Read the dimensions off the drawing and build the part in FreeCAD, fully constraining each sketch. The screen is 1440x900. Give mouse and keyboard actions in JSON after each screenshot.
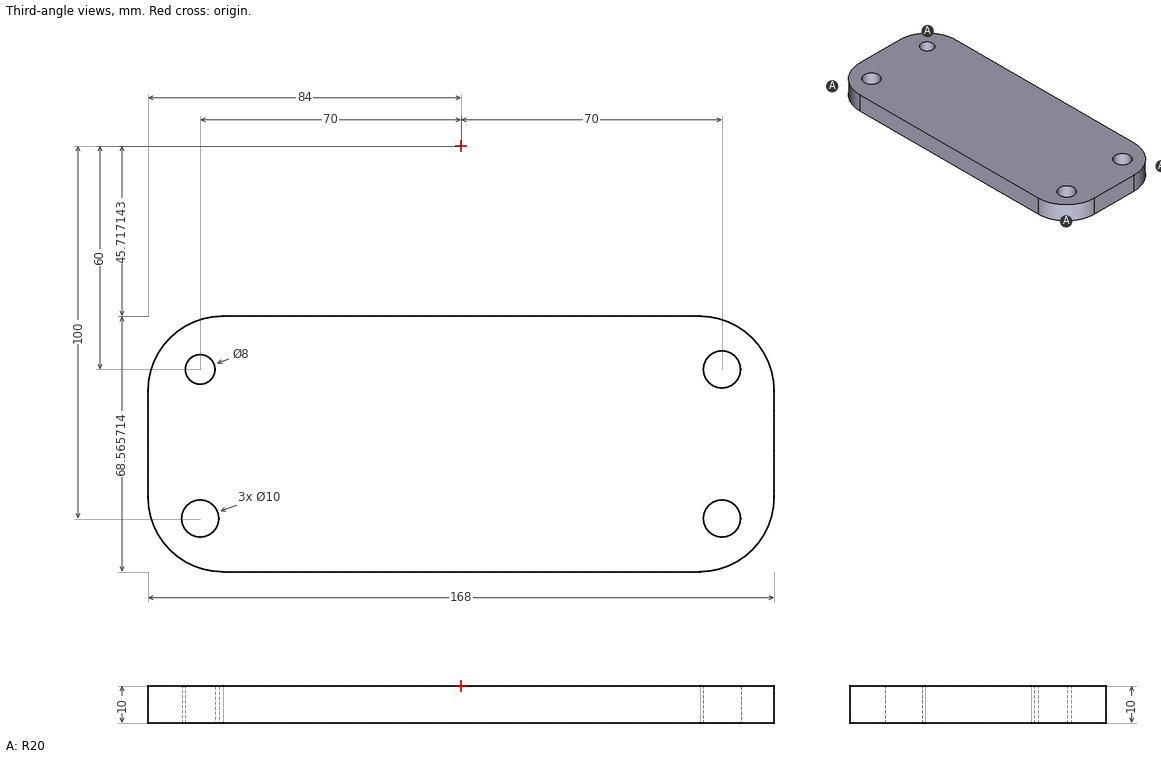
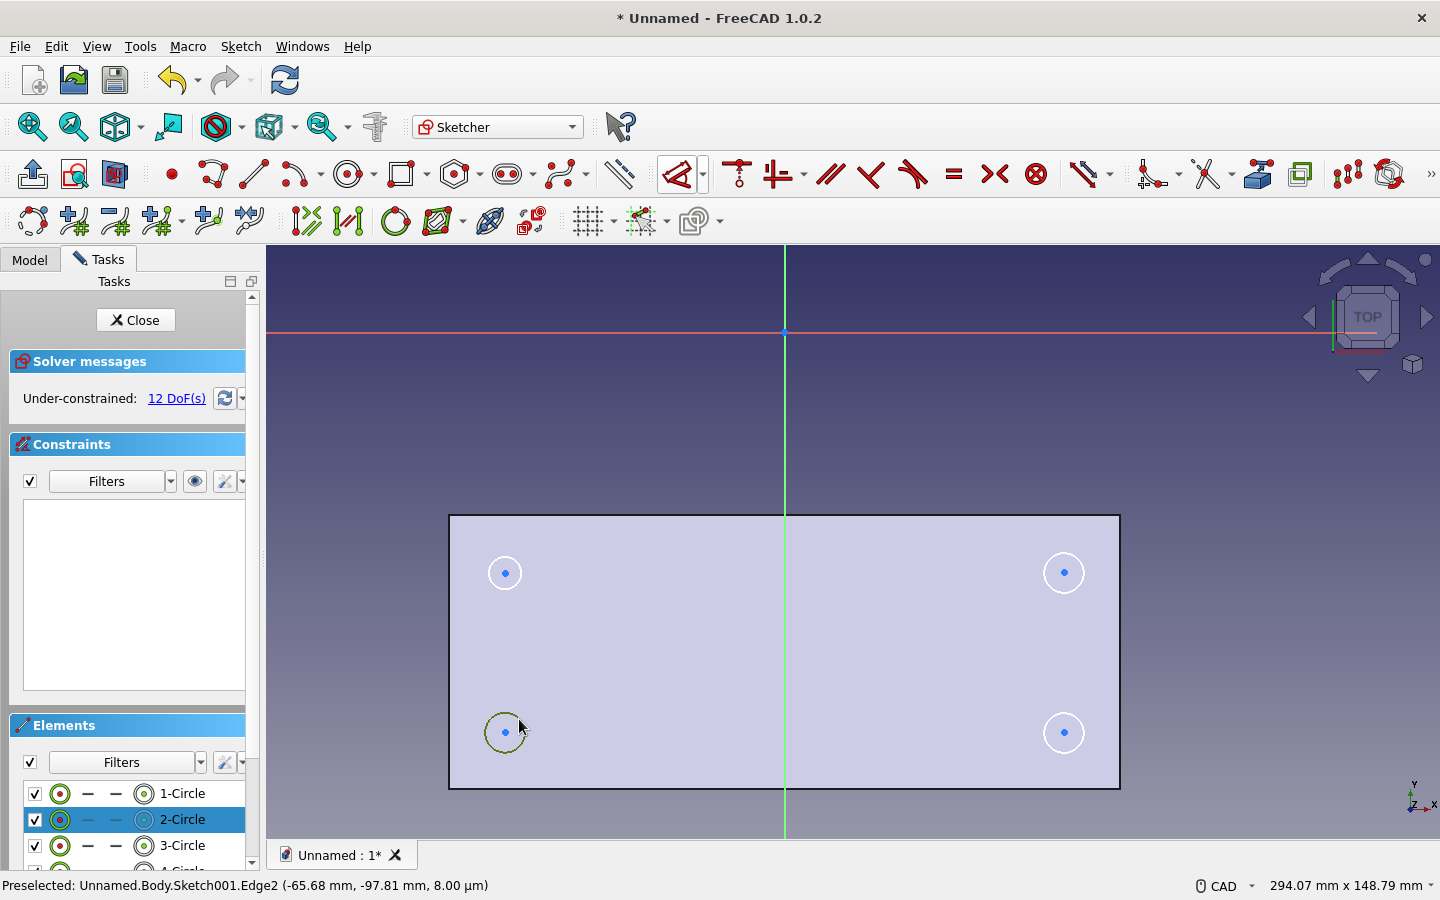
{"action": "left_click", "coordinate": [1078, 559]}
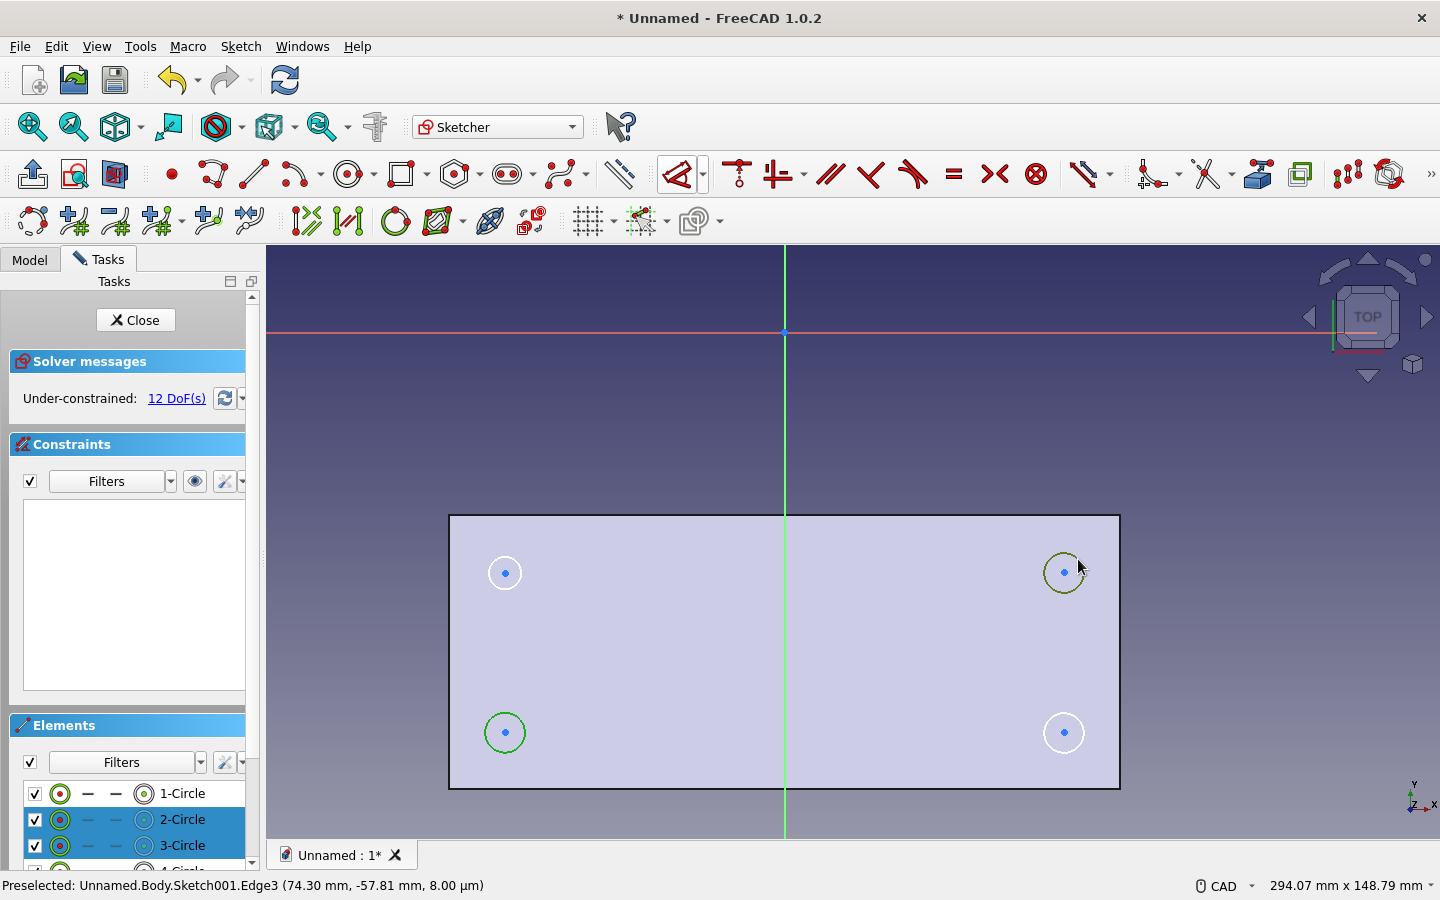
{"action": "left_click", "coordinate": [1078, 719]}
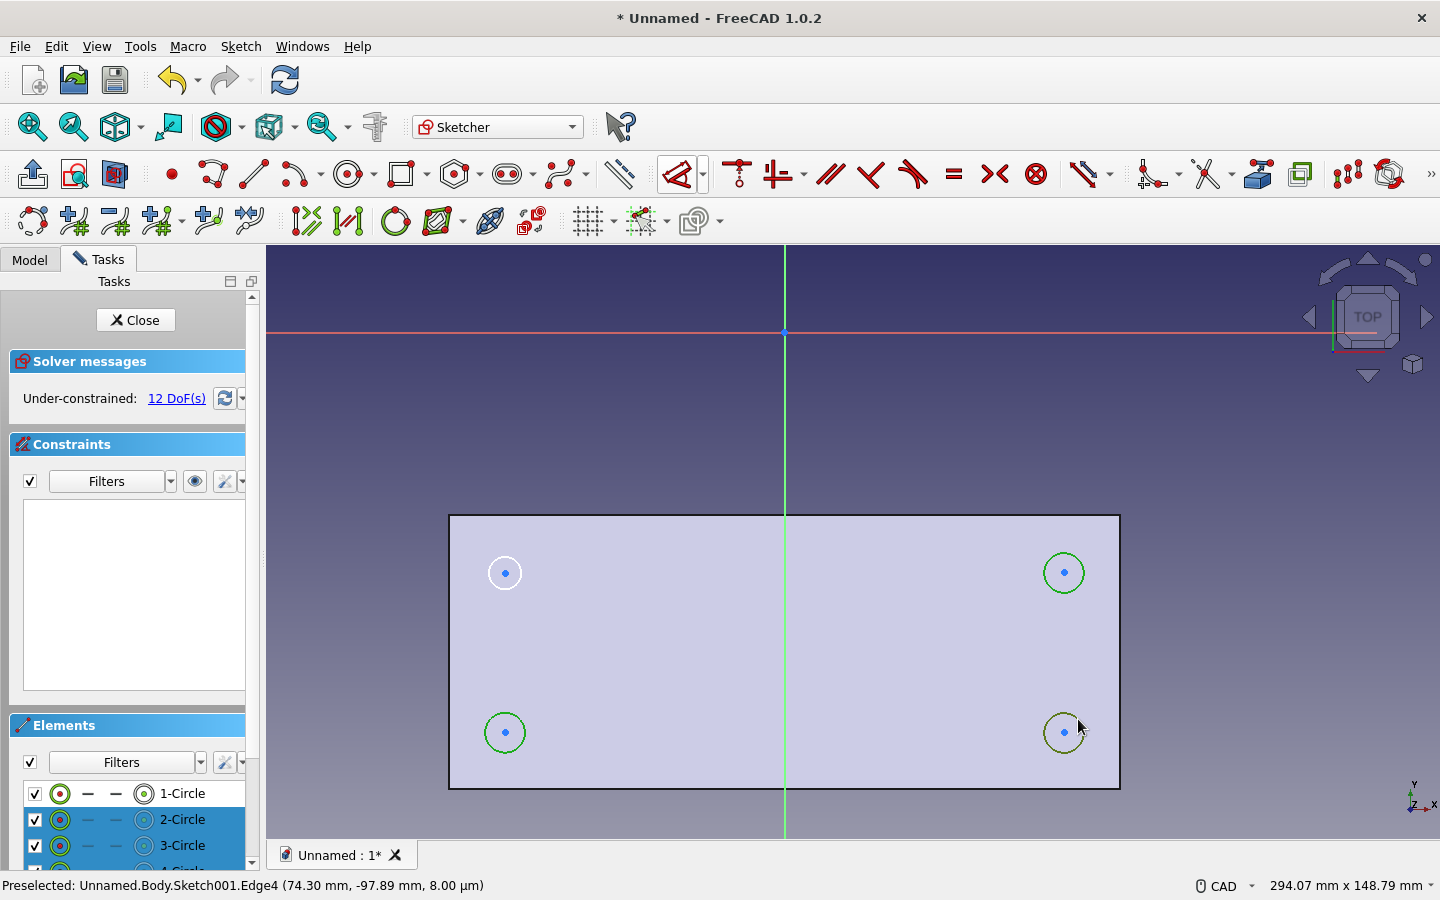
{"action": "left_click", "coordinate": [954, 174]}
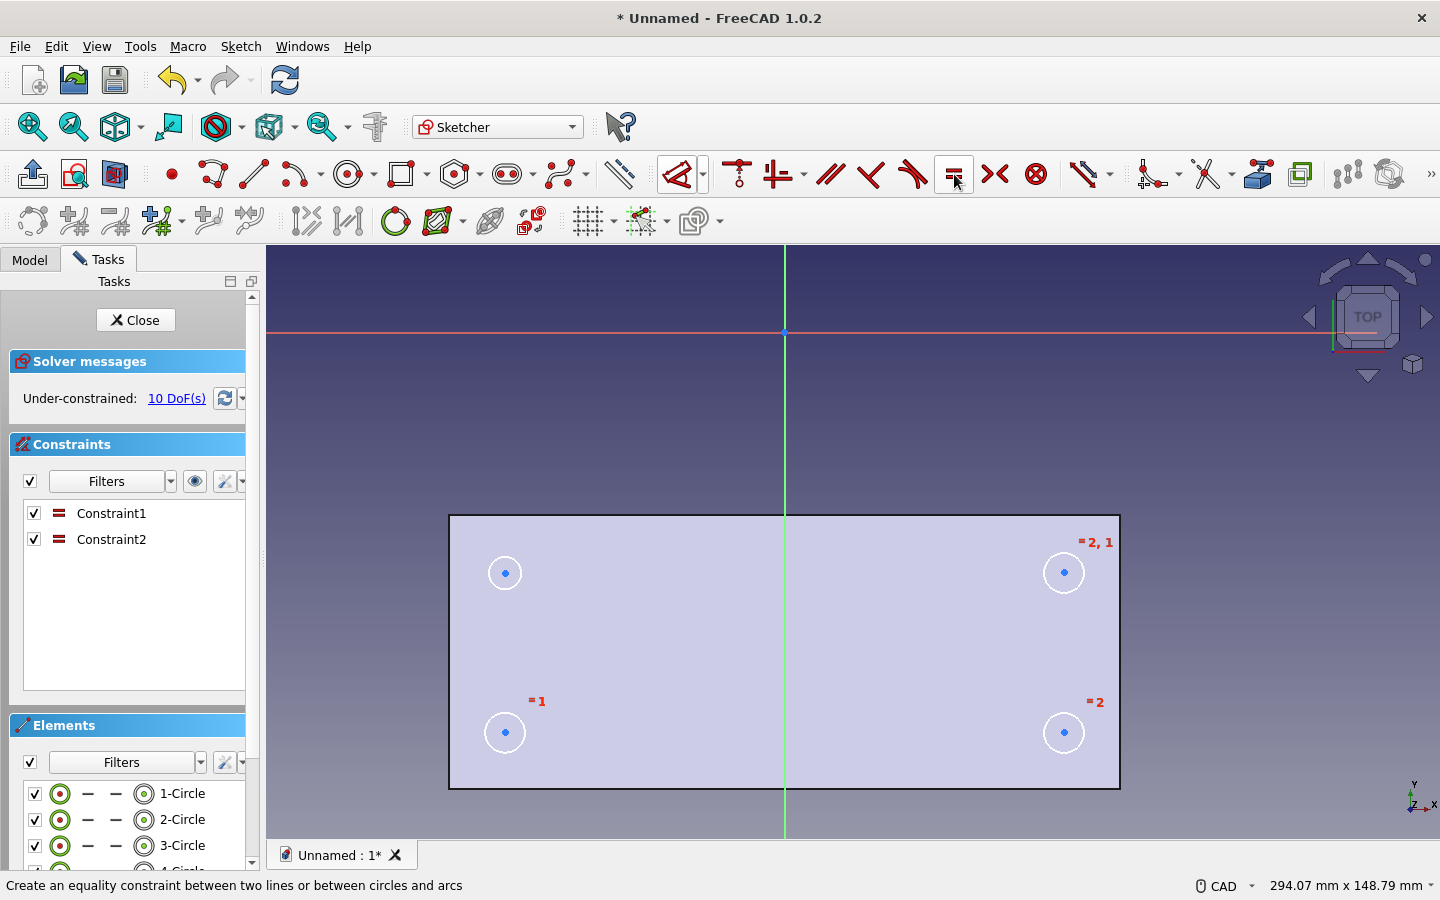
{"action": "left_click", "coordinate": [505, 573]}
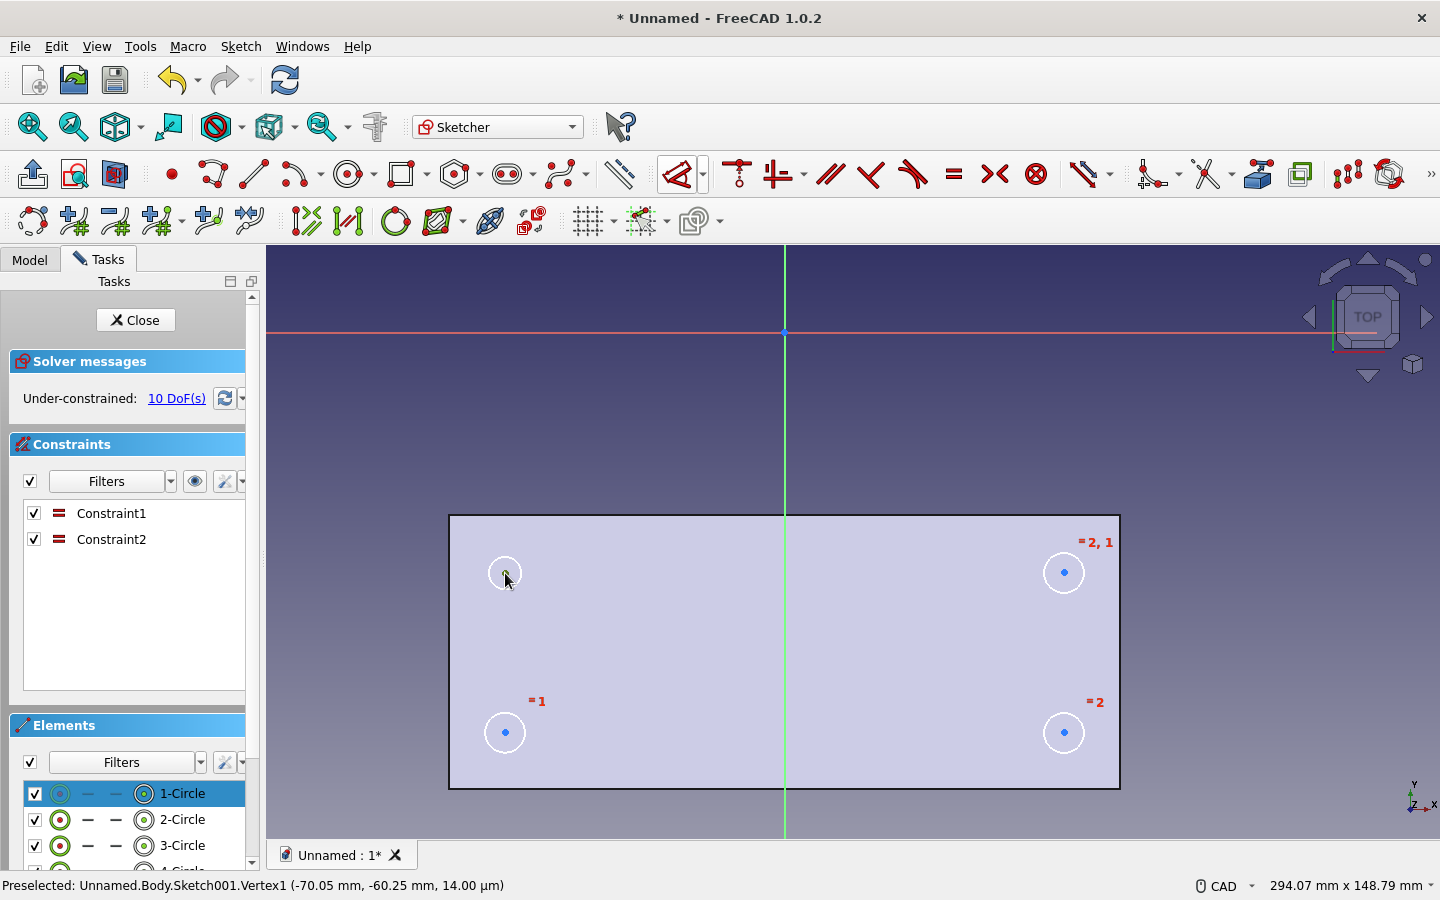
{"action": "left_click", "coordinate": [505, 733]}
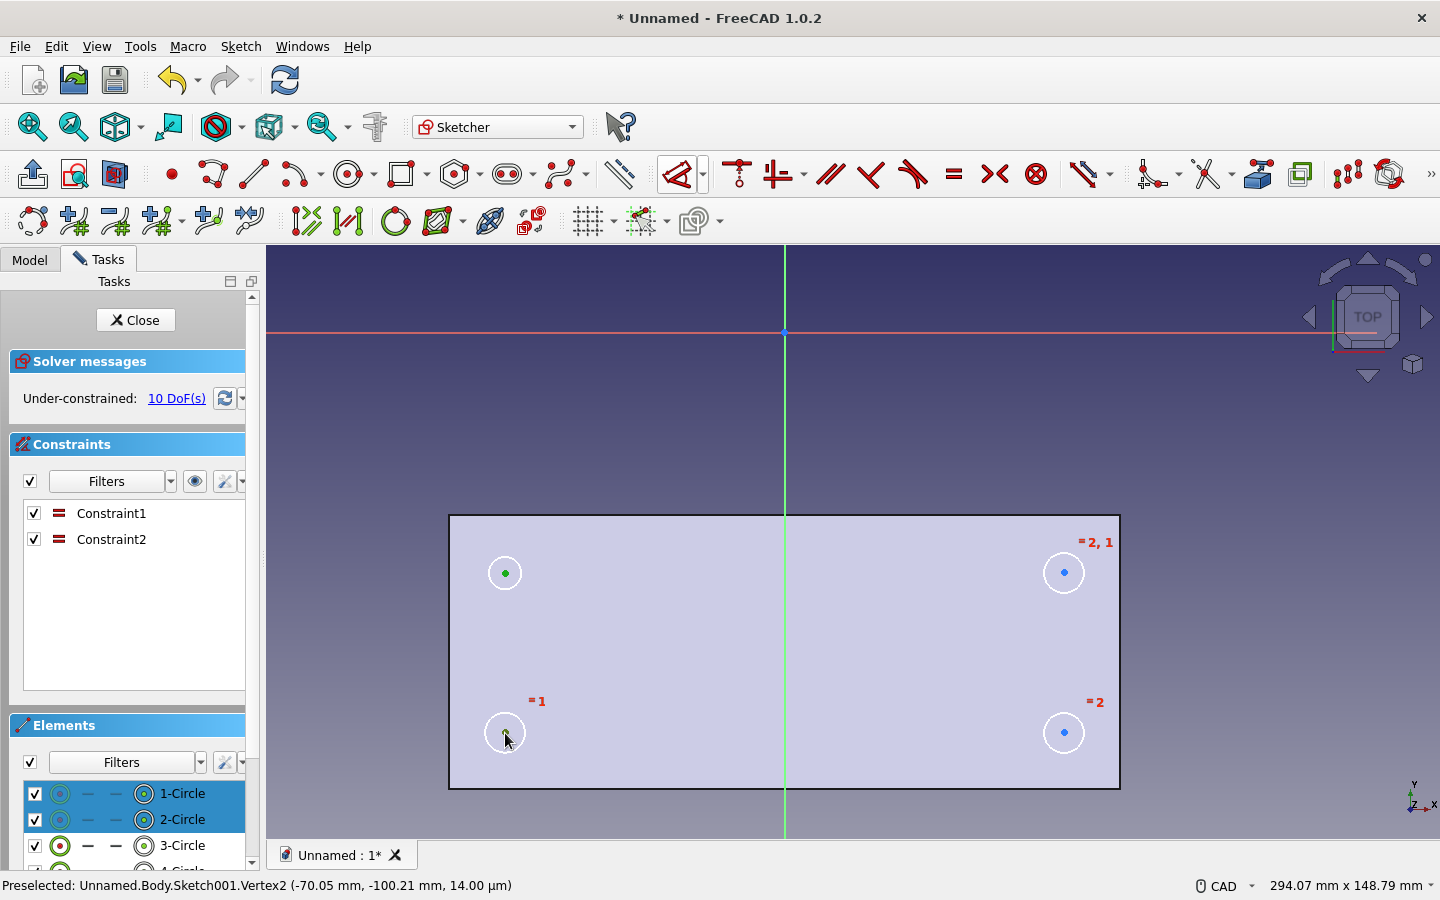
{"action": "key", "text": "v"}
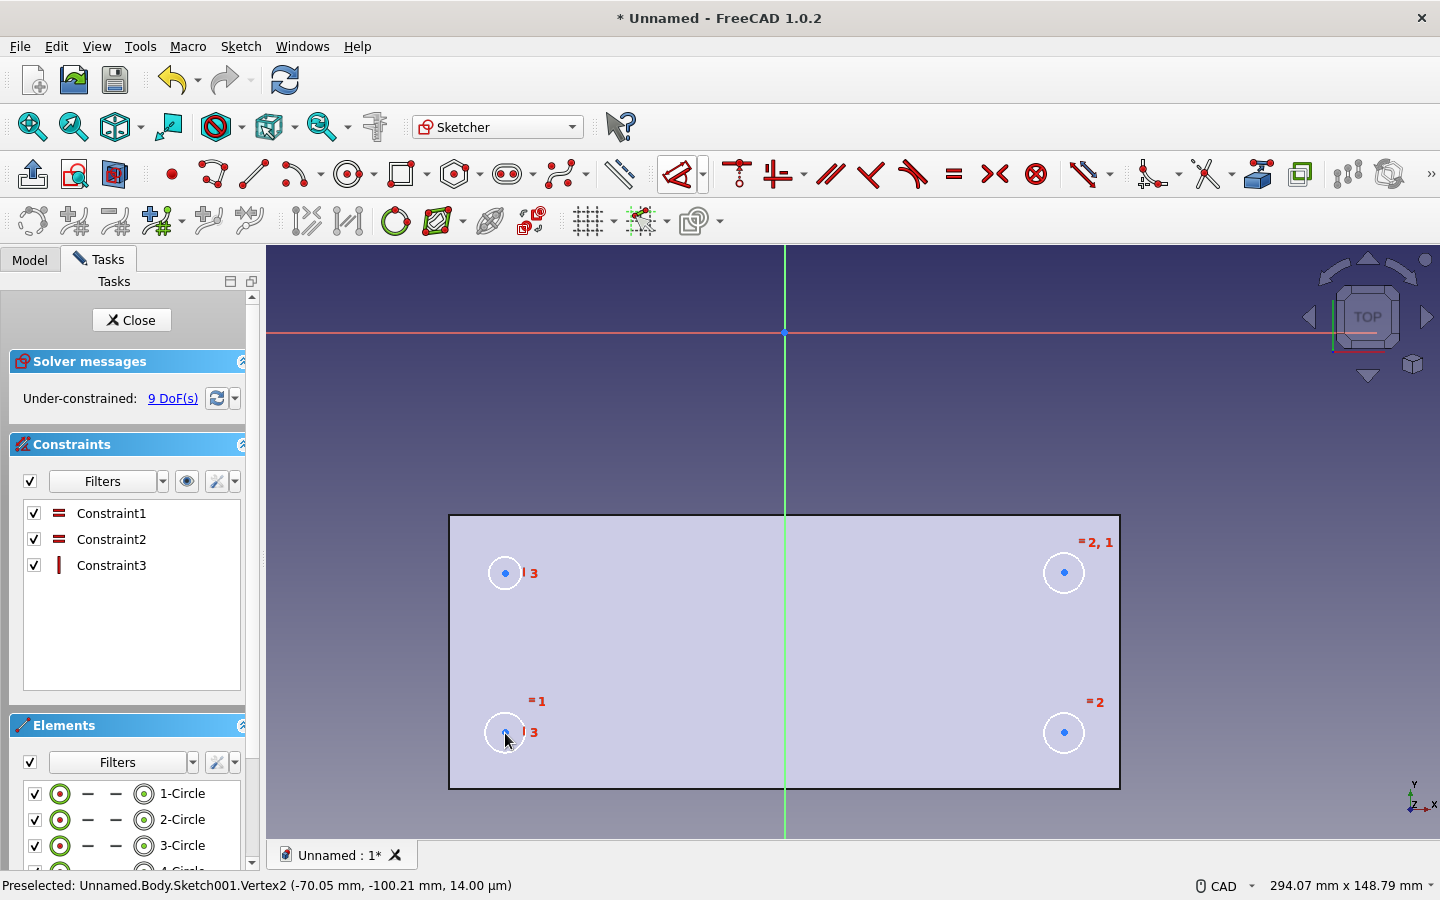
{"action": "left_click", "coordinate": [505, 573]}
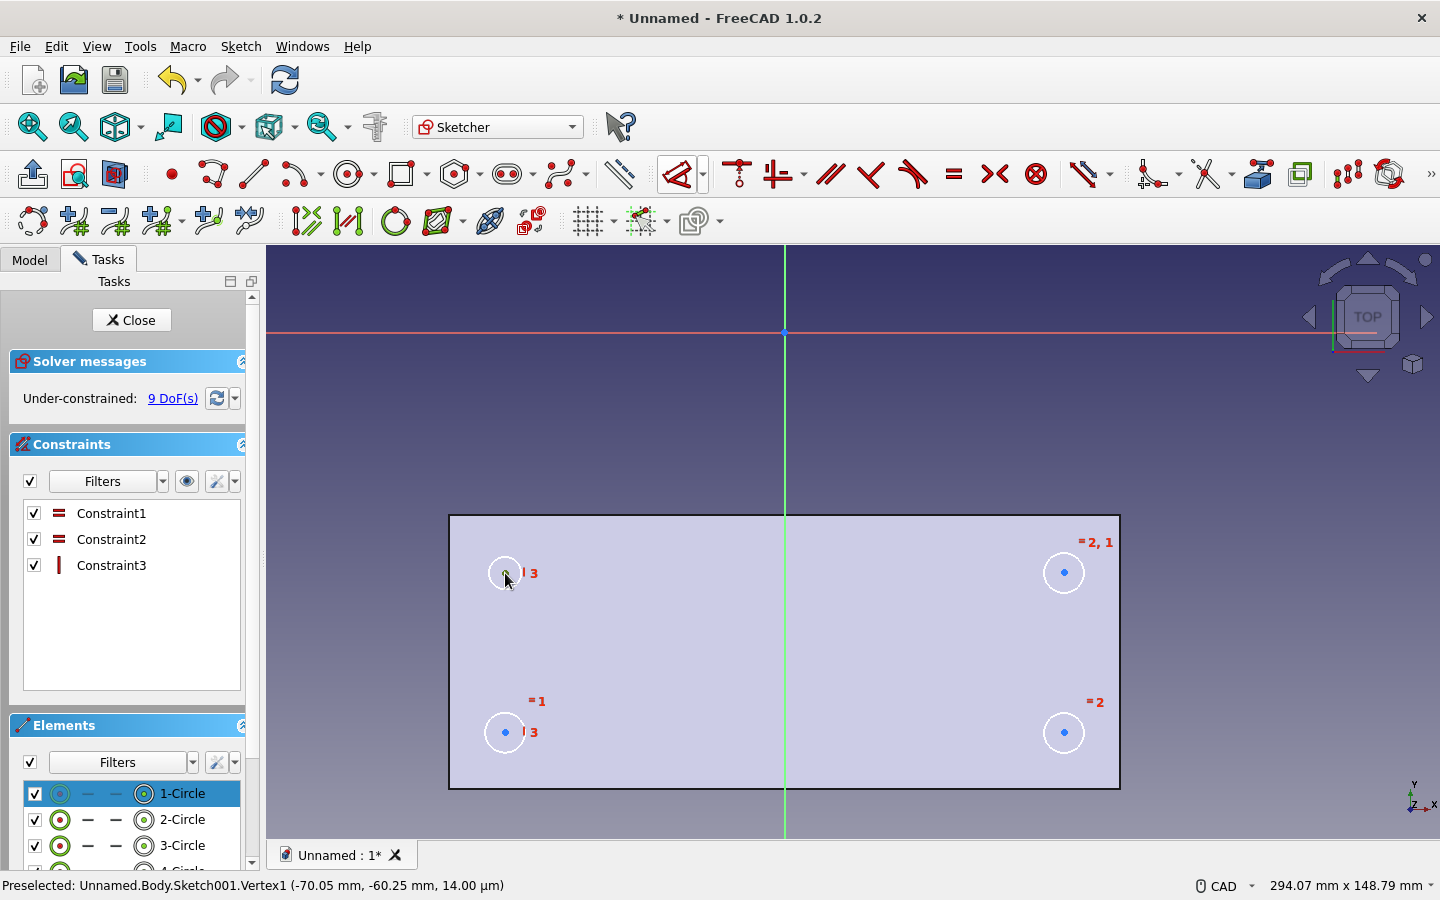
{"action": "left_click", "coordinate": [1064, 573]}